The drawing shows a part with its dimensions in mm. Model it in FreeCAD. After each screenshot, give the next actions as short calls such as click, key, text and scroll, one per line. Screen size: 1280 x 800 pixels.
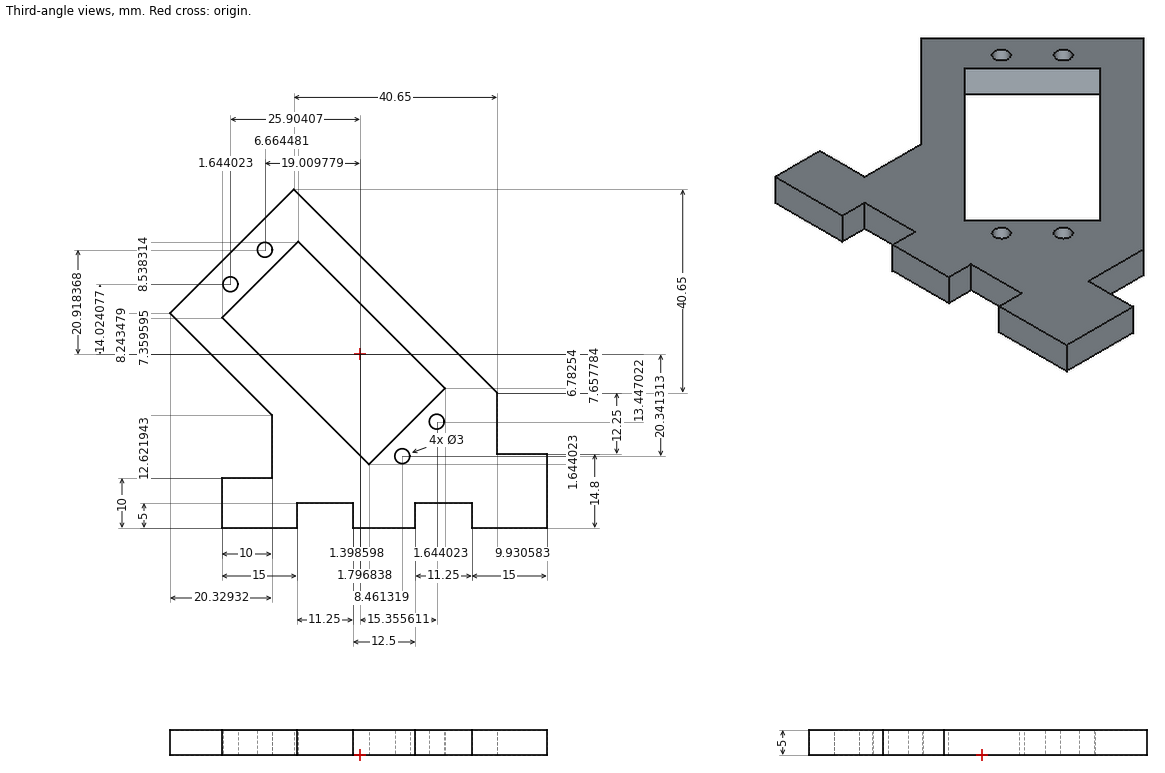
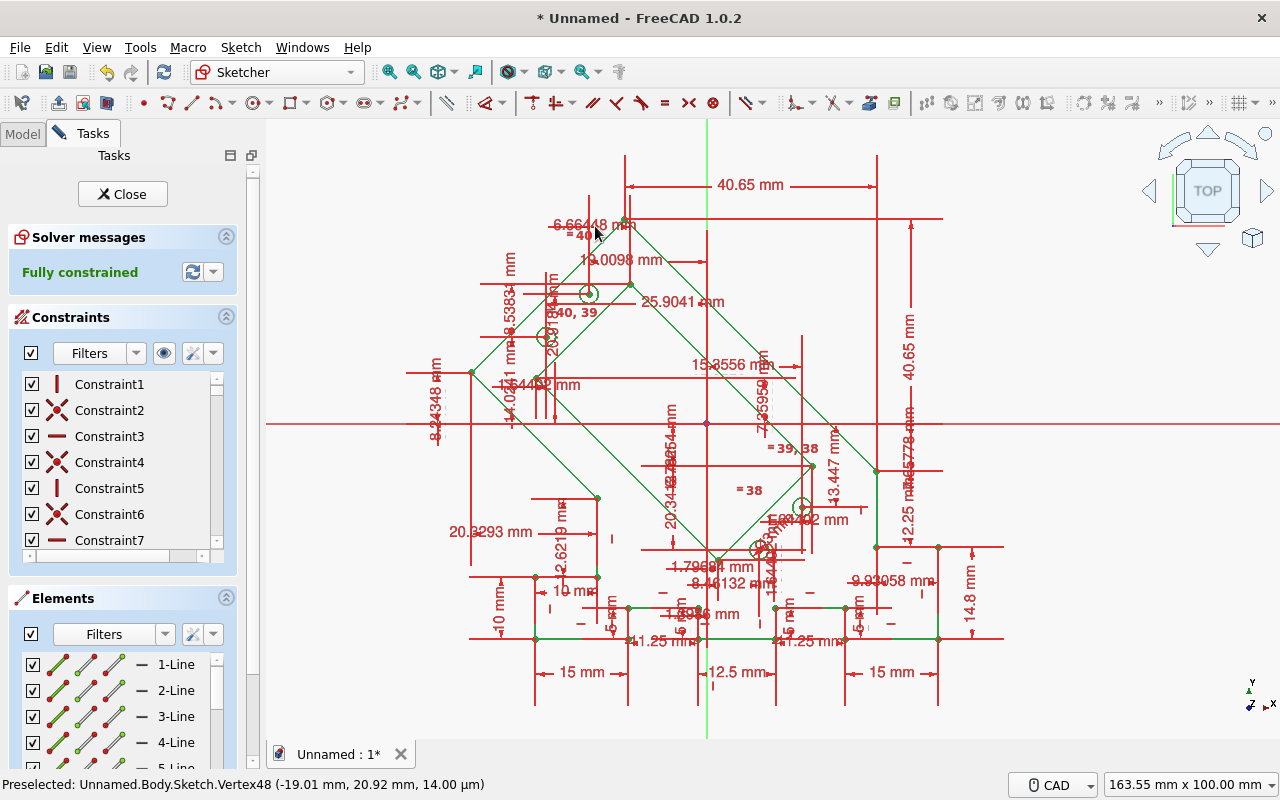
click(123, 194)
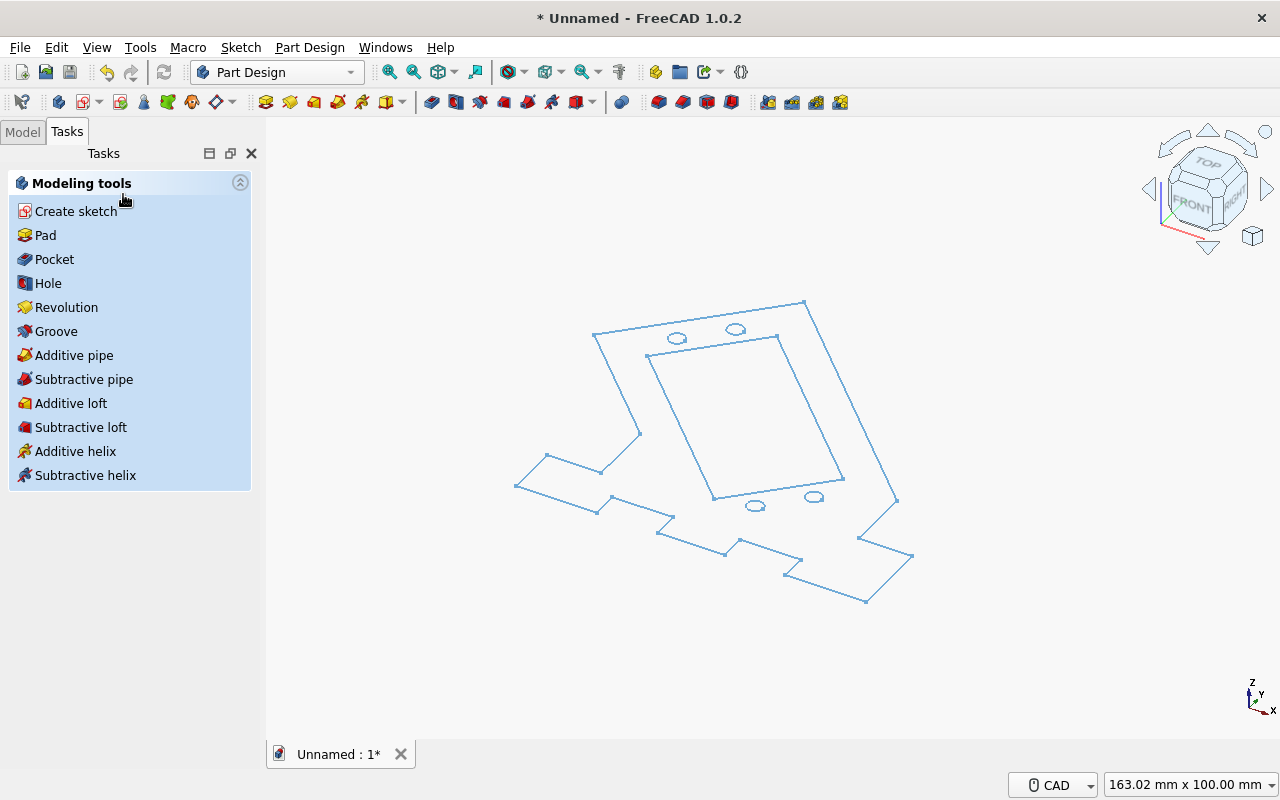
click(266, 102)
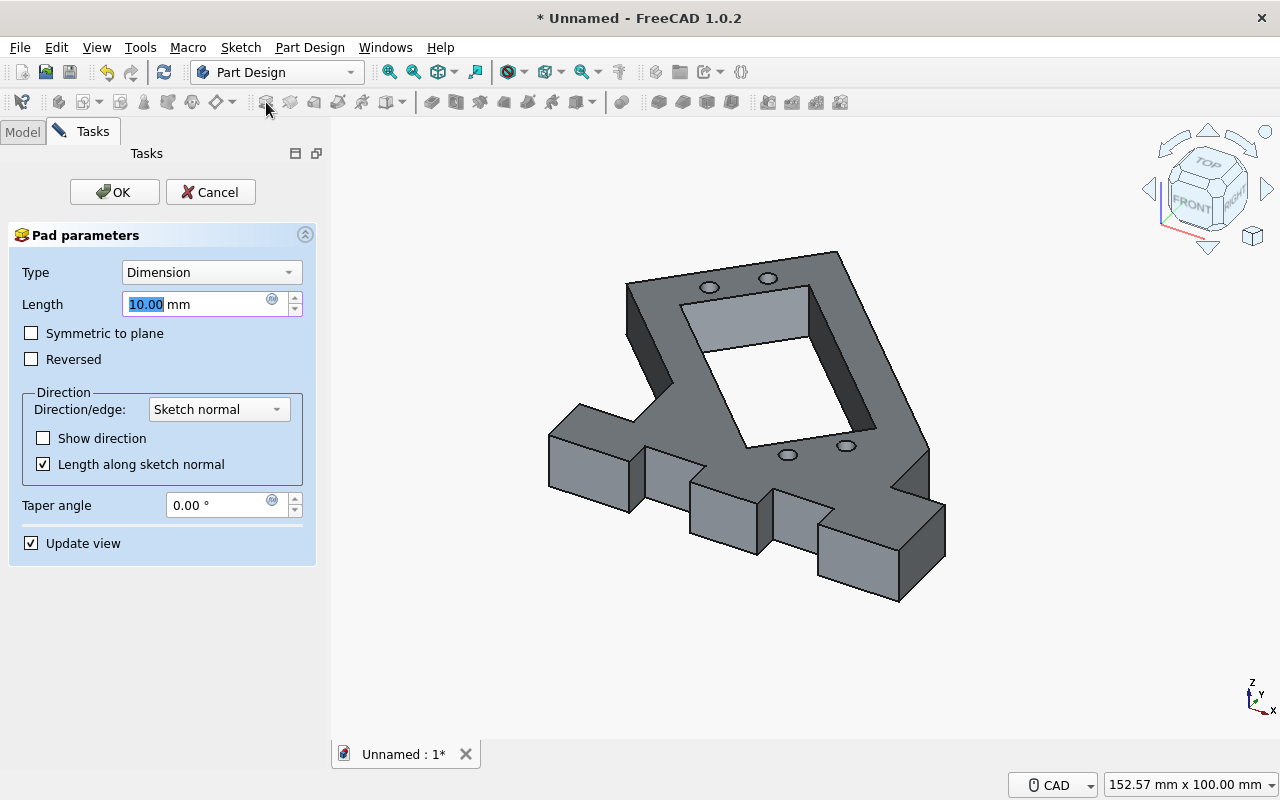
text(5)
key(Tab)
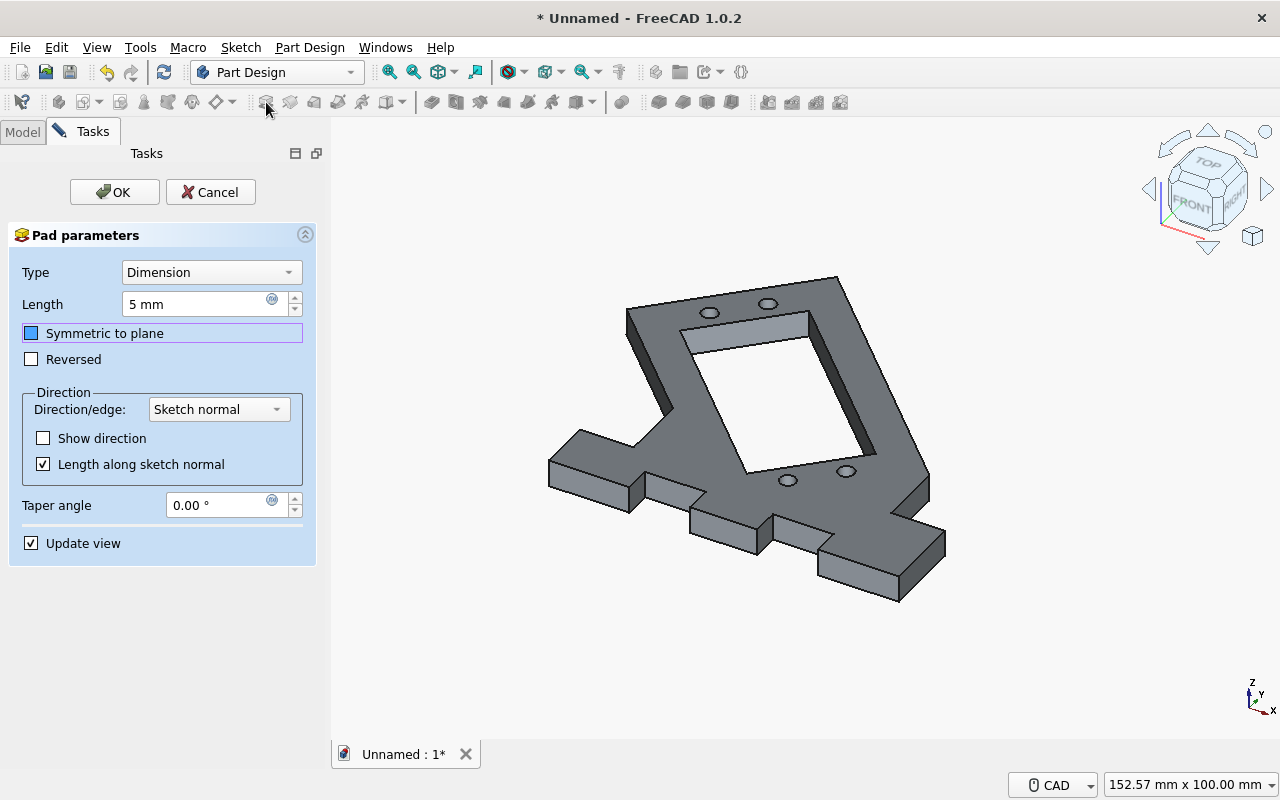
click(115, 192)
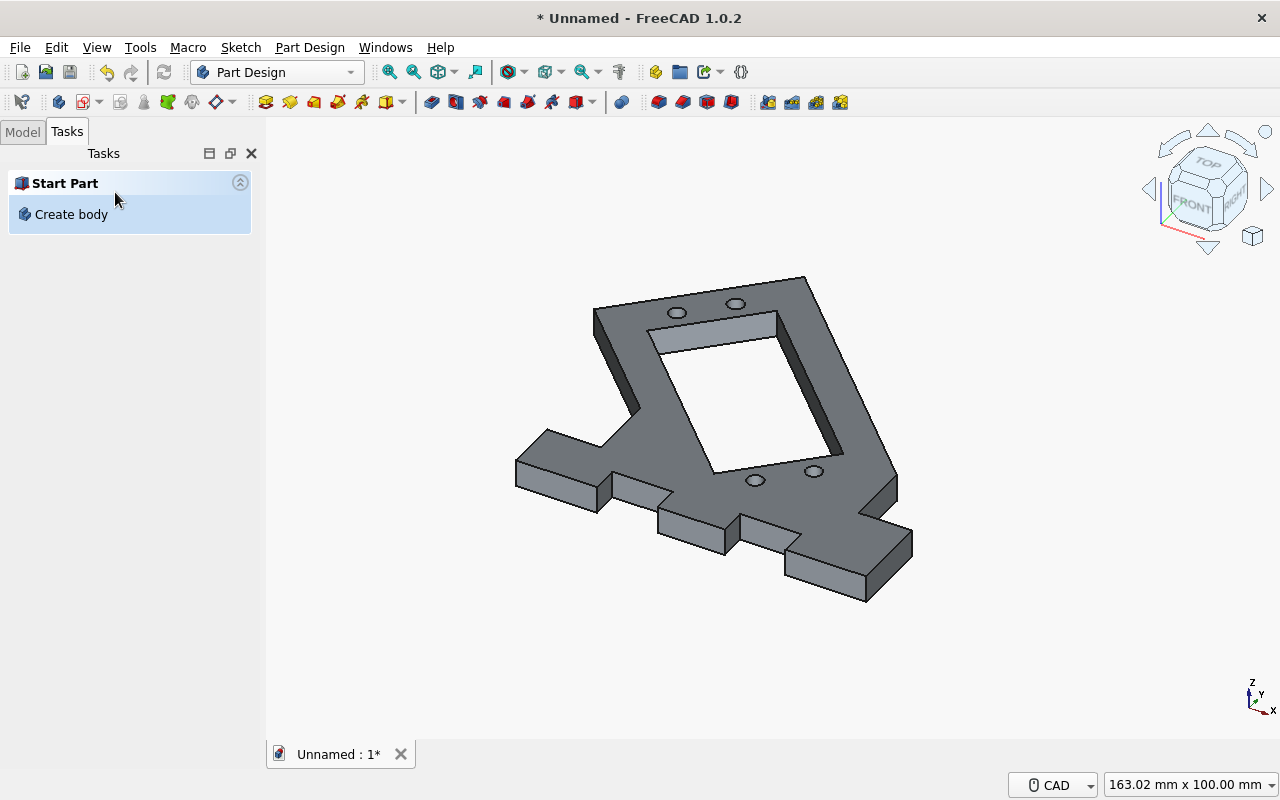
key(0)